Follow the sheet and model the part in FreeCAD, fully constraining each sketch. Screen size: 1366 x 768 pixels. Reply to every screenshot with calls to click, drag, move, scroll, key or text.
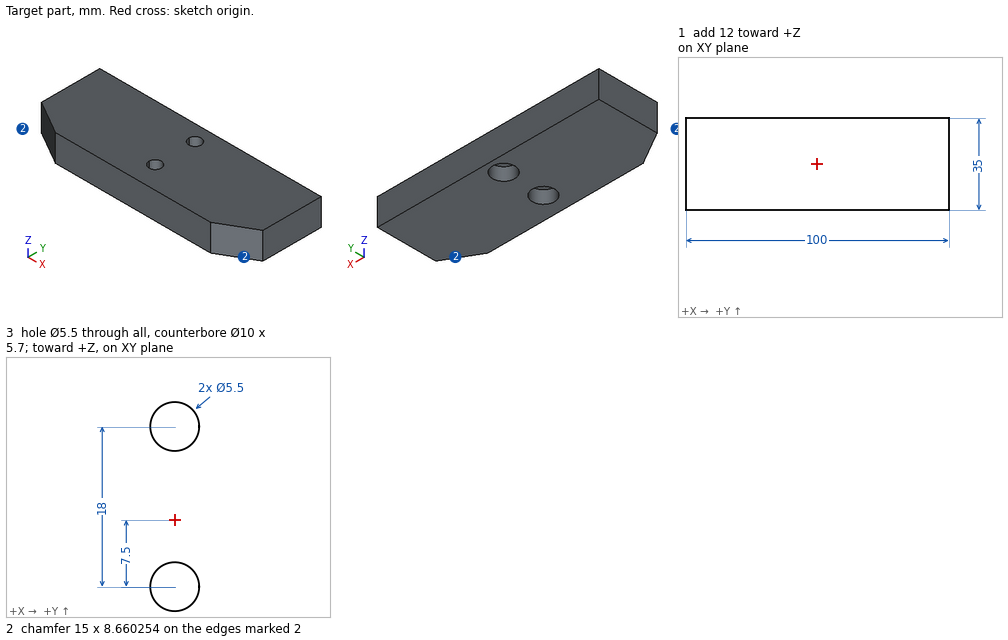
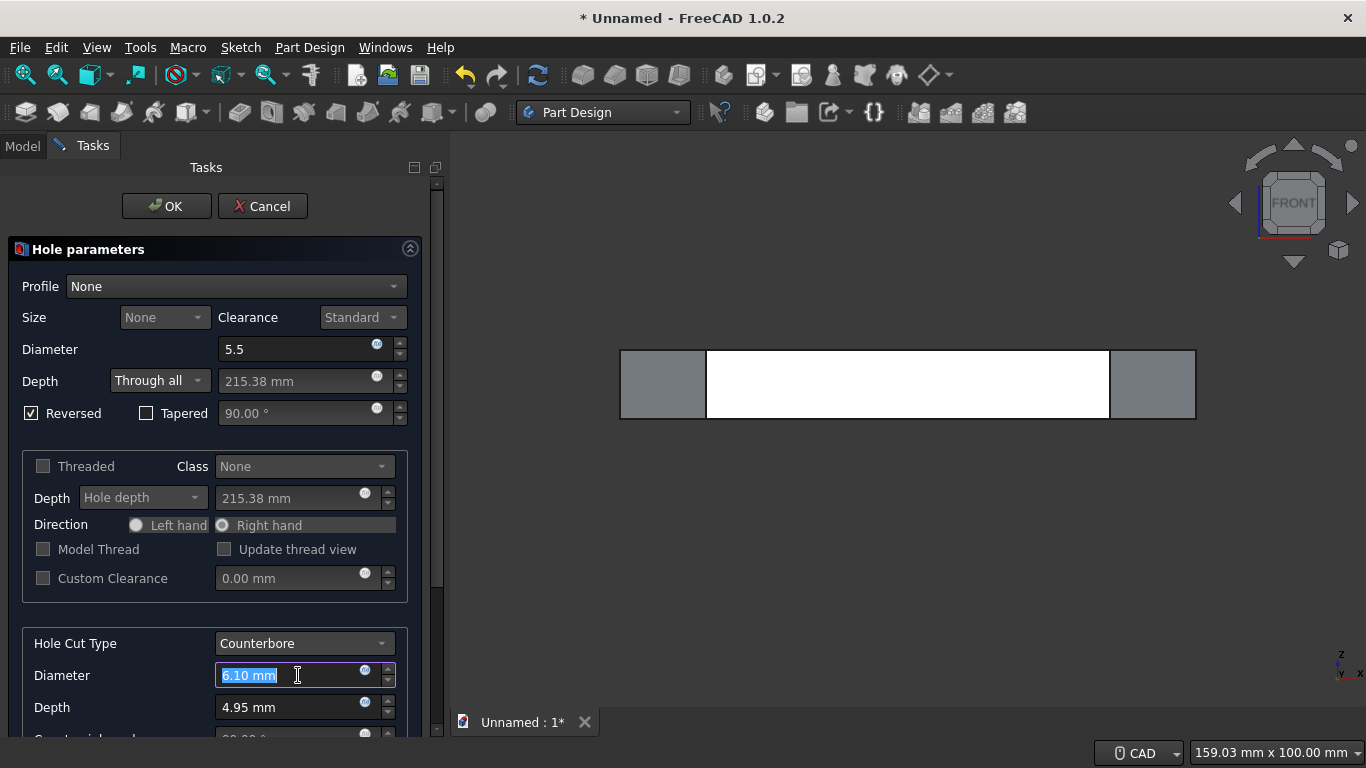
text(10)
key(Tab)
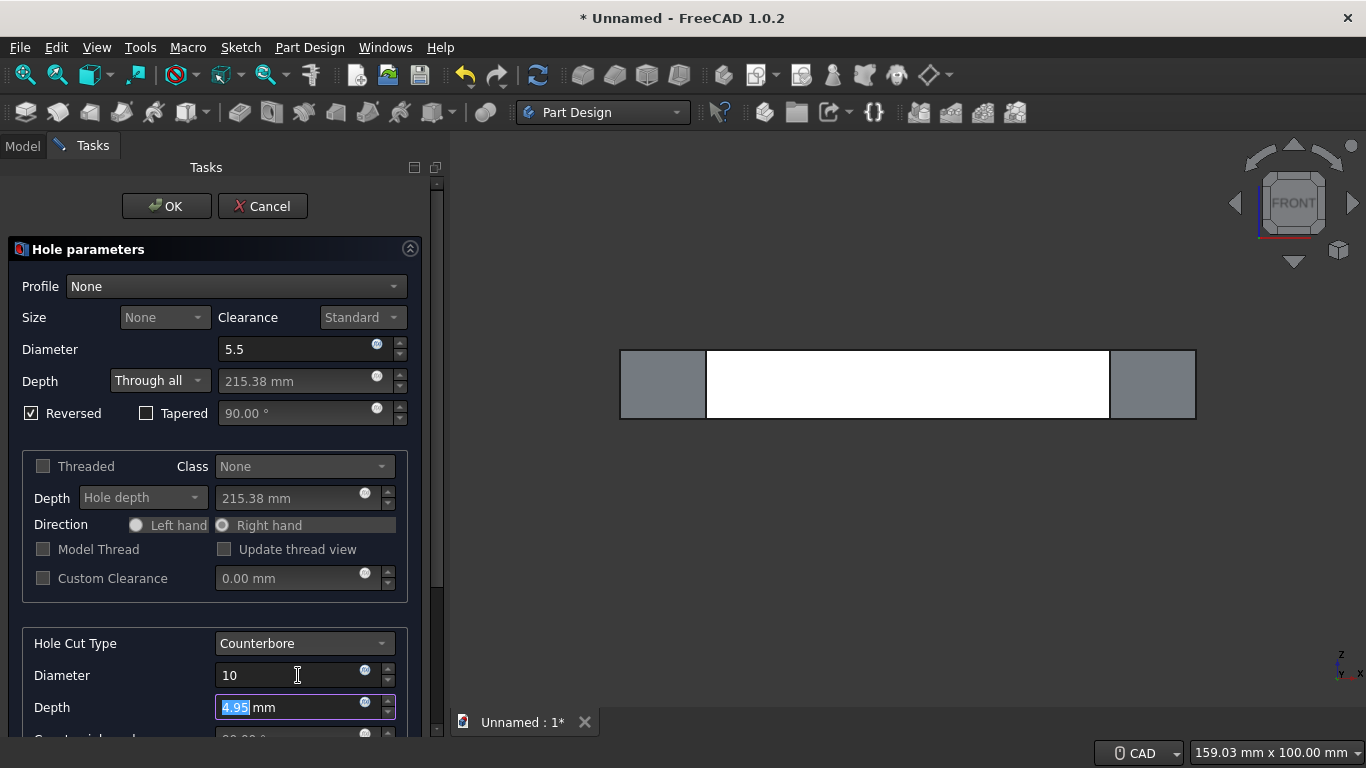
text(5.7)
key(Tab)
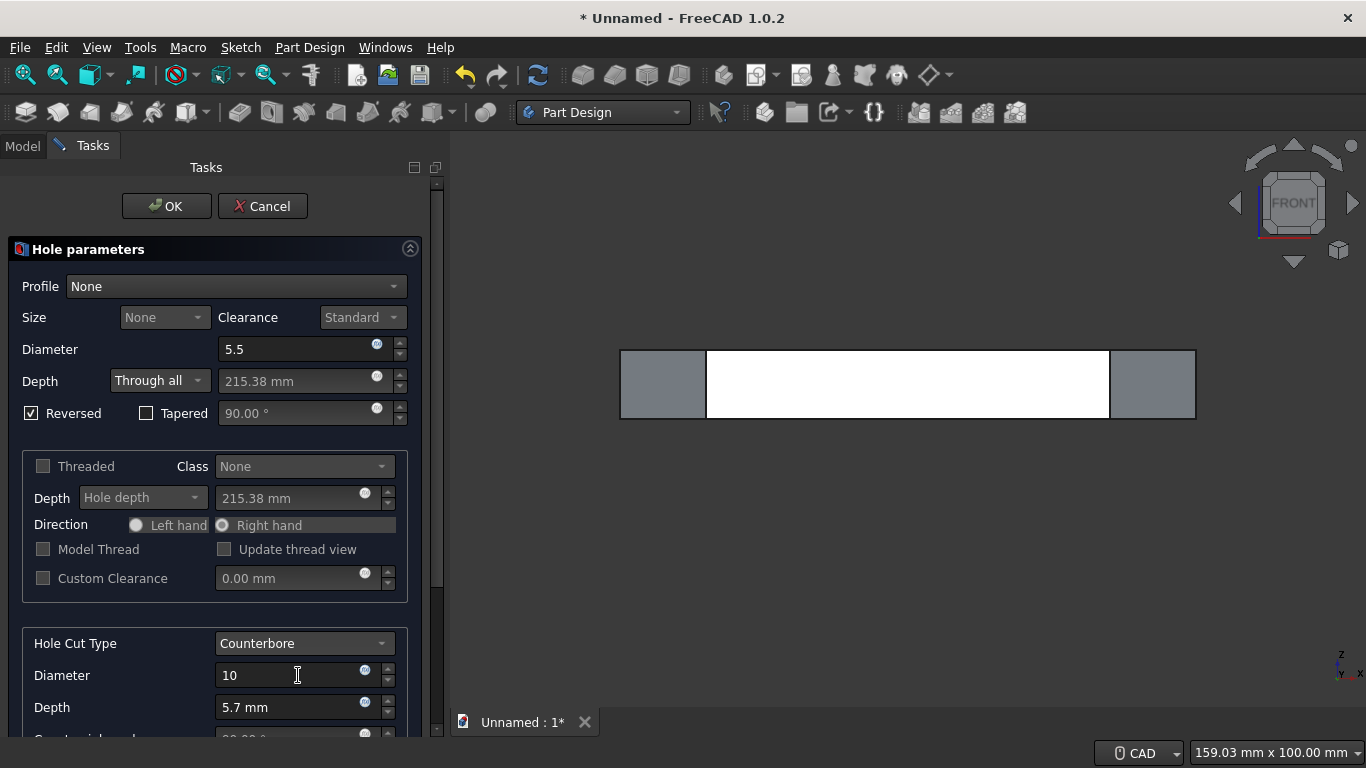
click(167, 206)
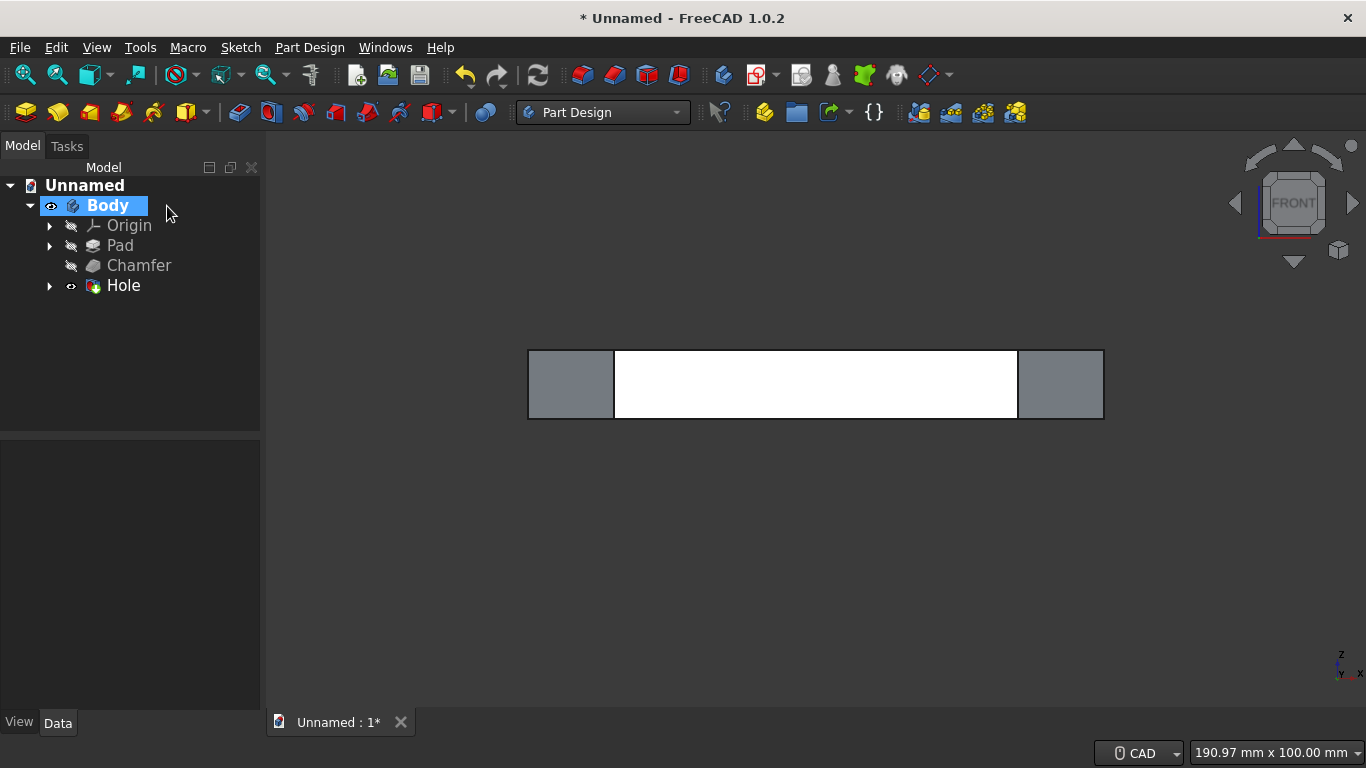
key(0)